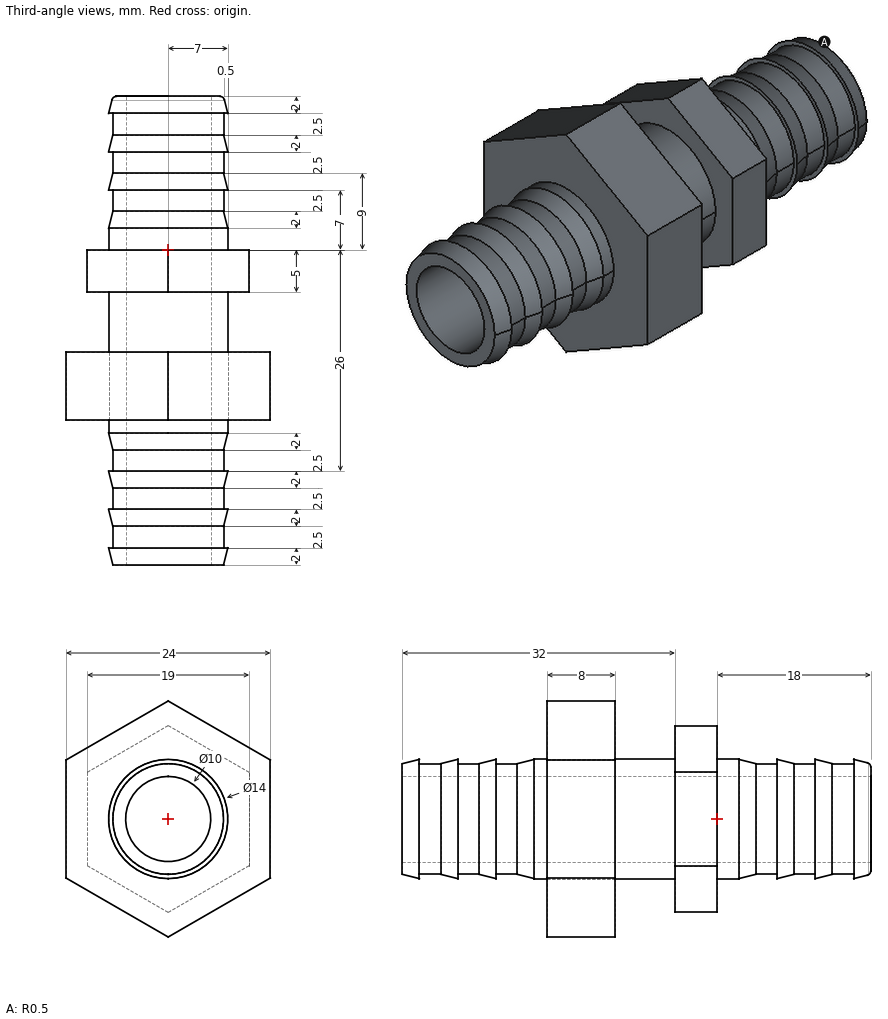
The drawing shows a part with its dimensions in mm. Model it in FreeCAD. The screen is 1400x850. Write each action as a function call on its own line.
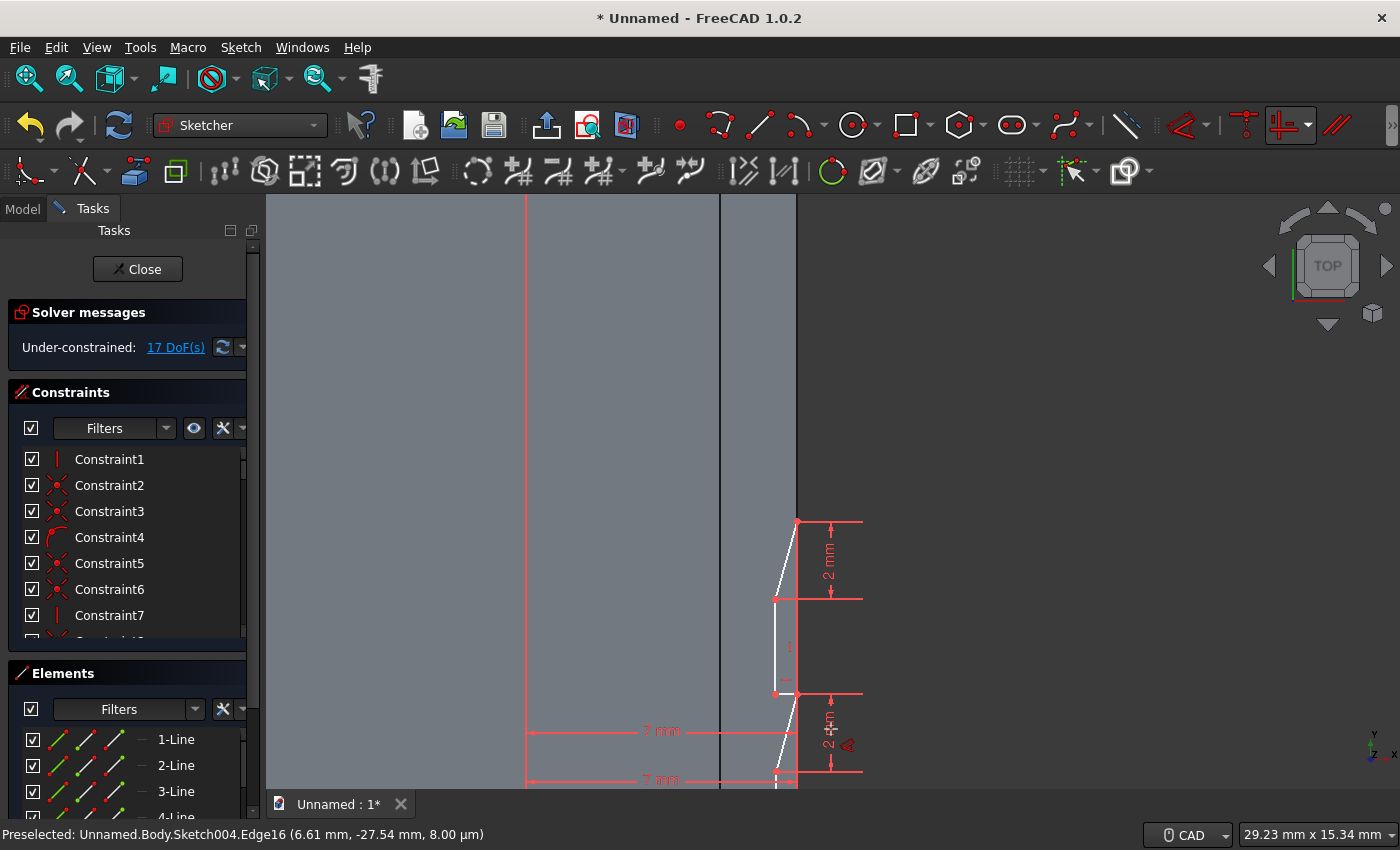
scroll(785, 579, down, 9)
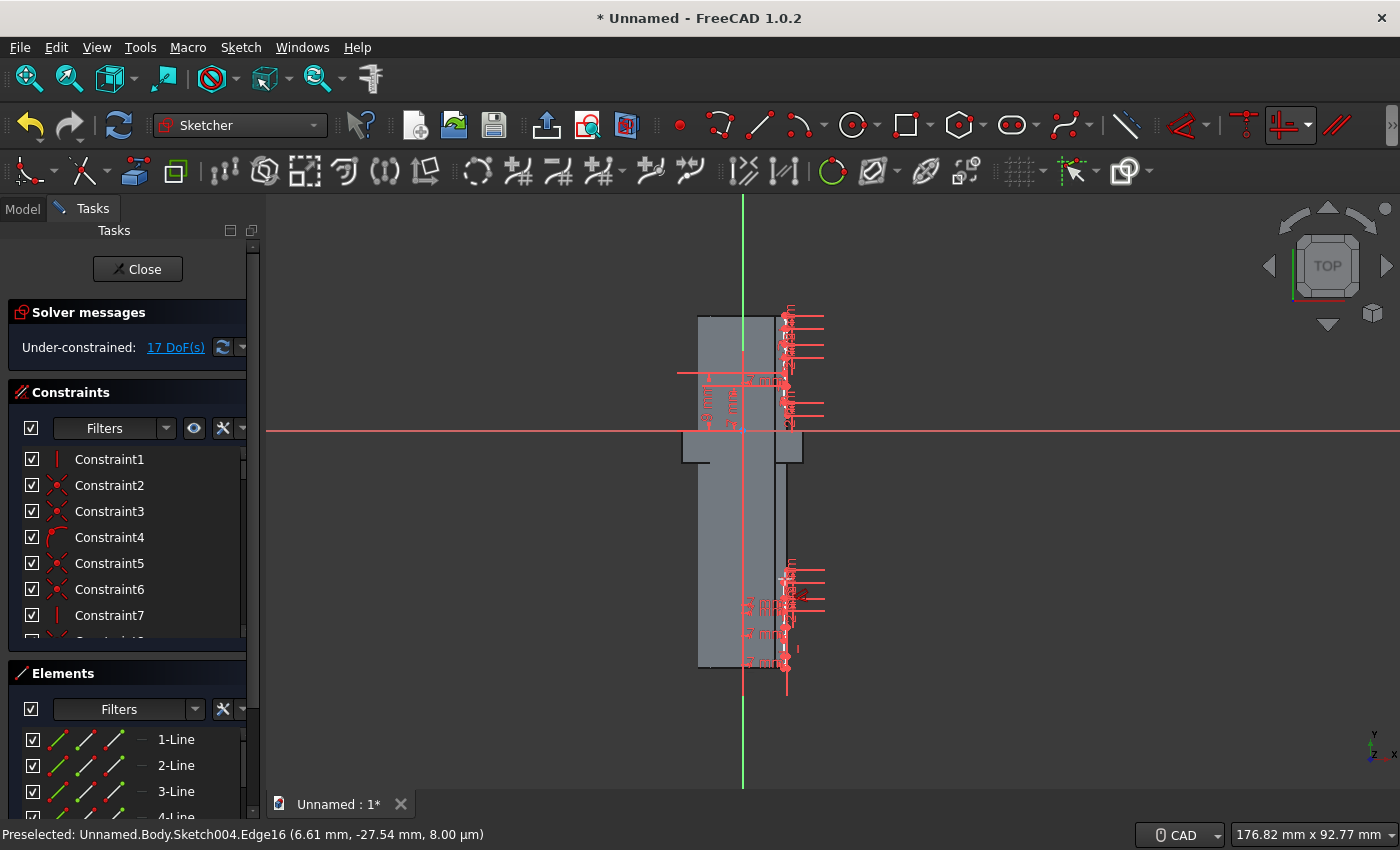
scroll(785, 636, up, 9)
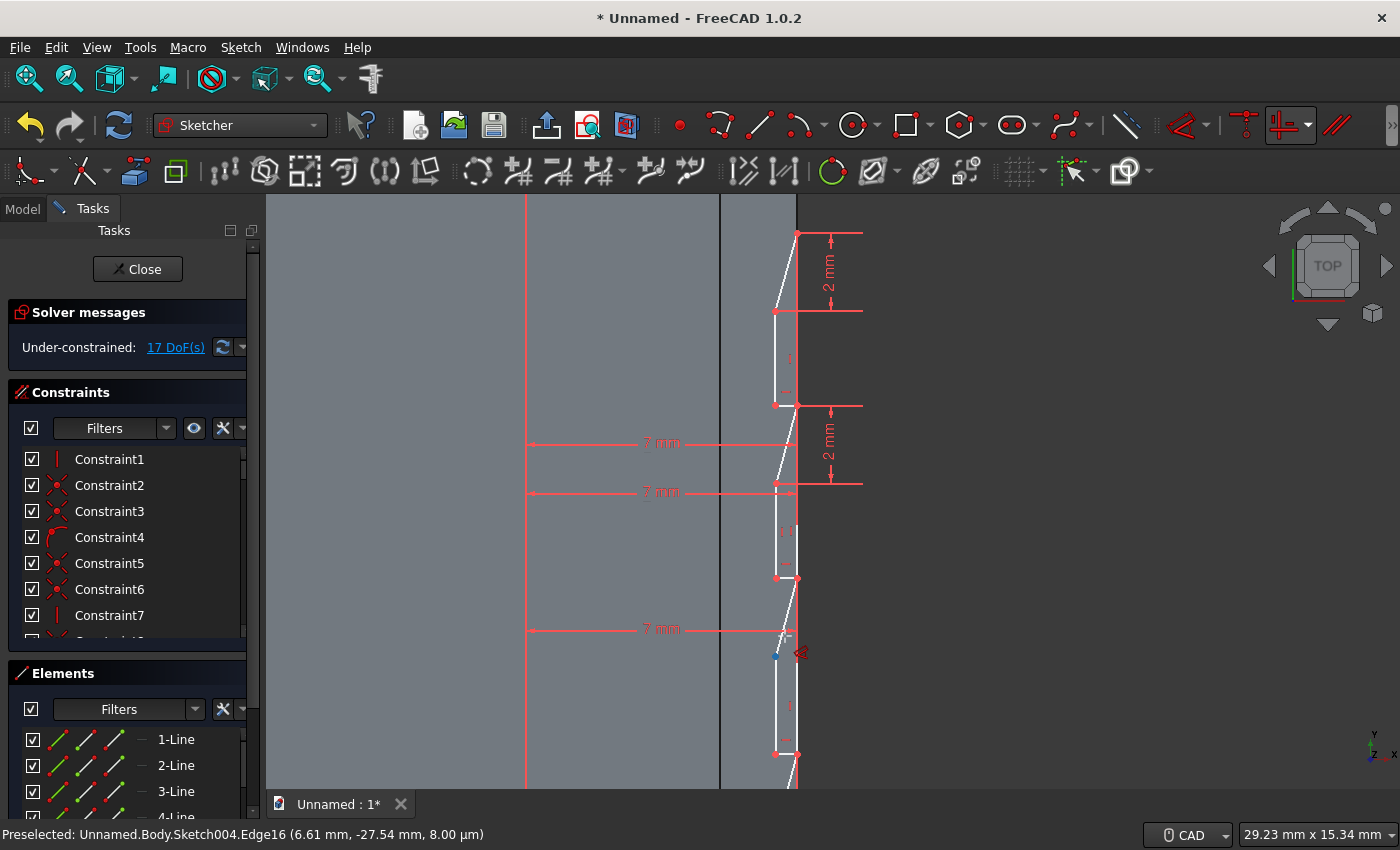
click(782, 633)
click(831, 617)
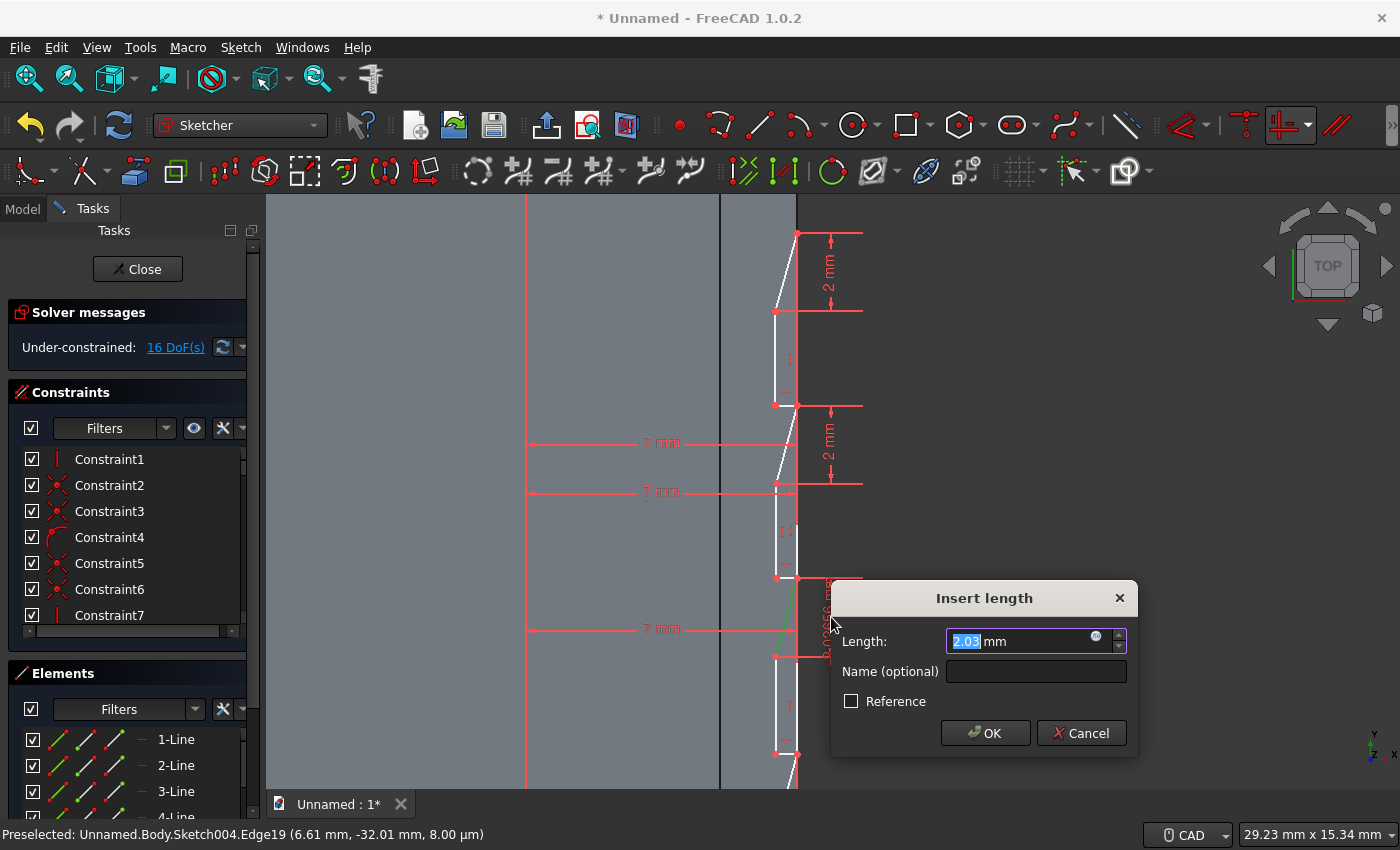
text(2)
key(Return)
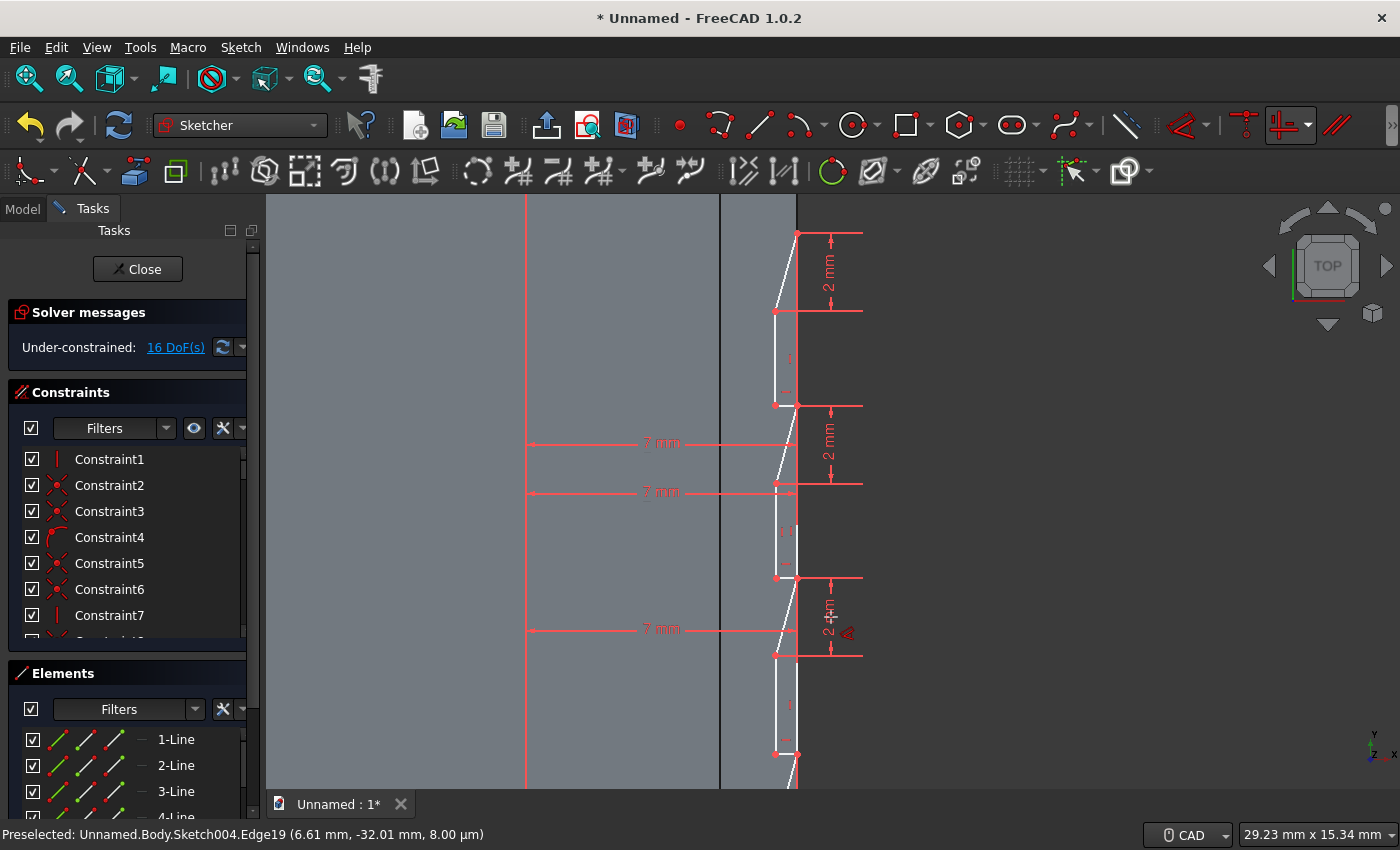
scroll(785, 636, down, 9)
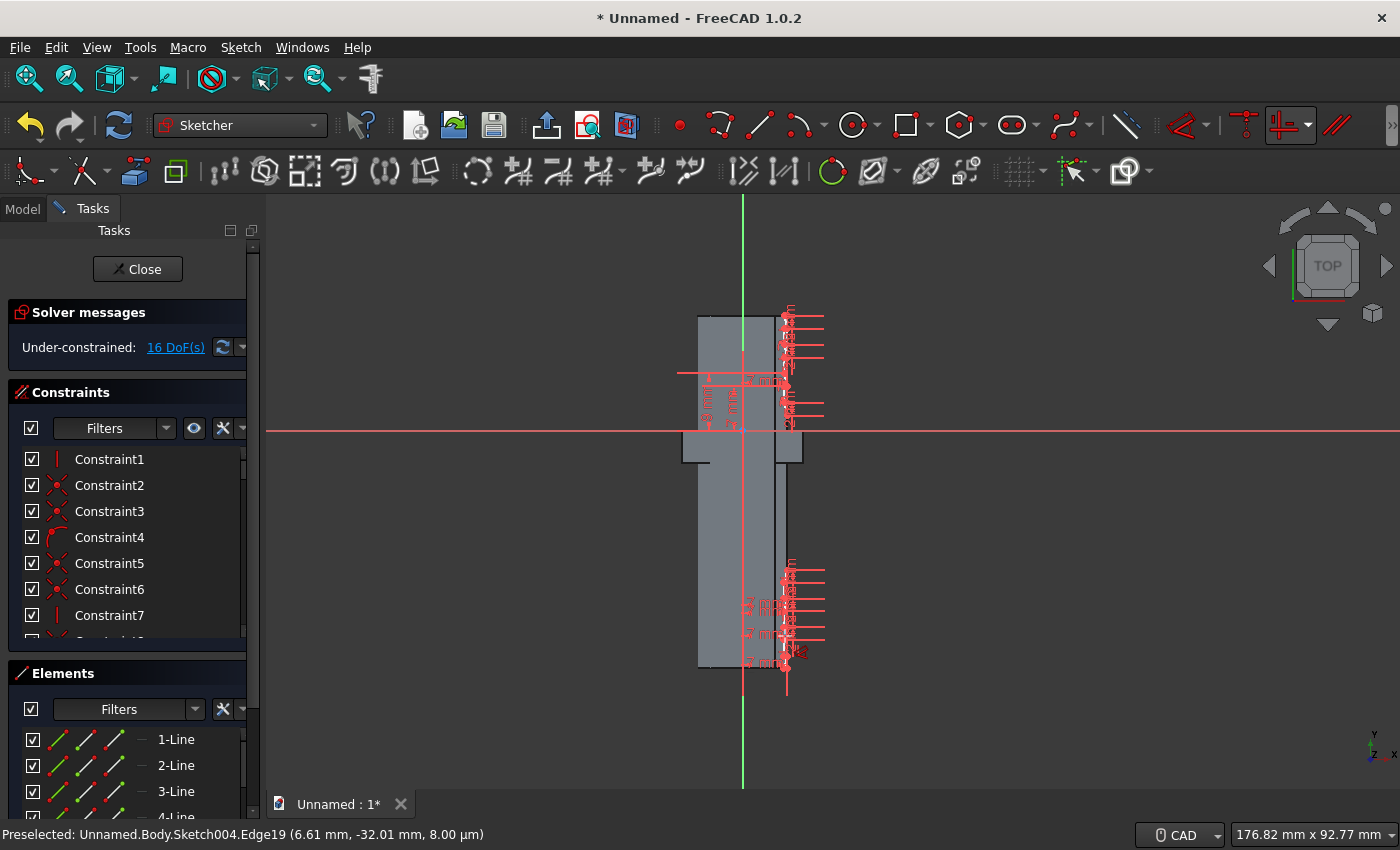
scroll(785, 665, up, 9)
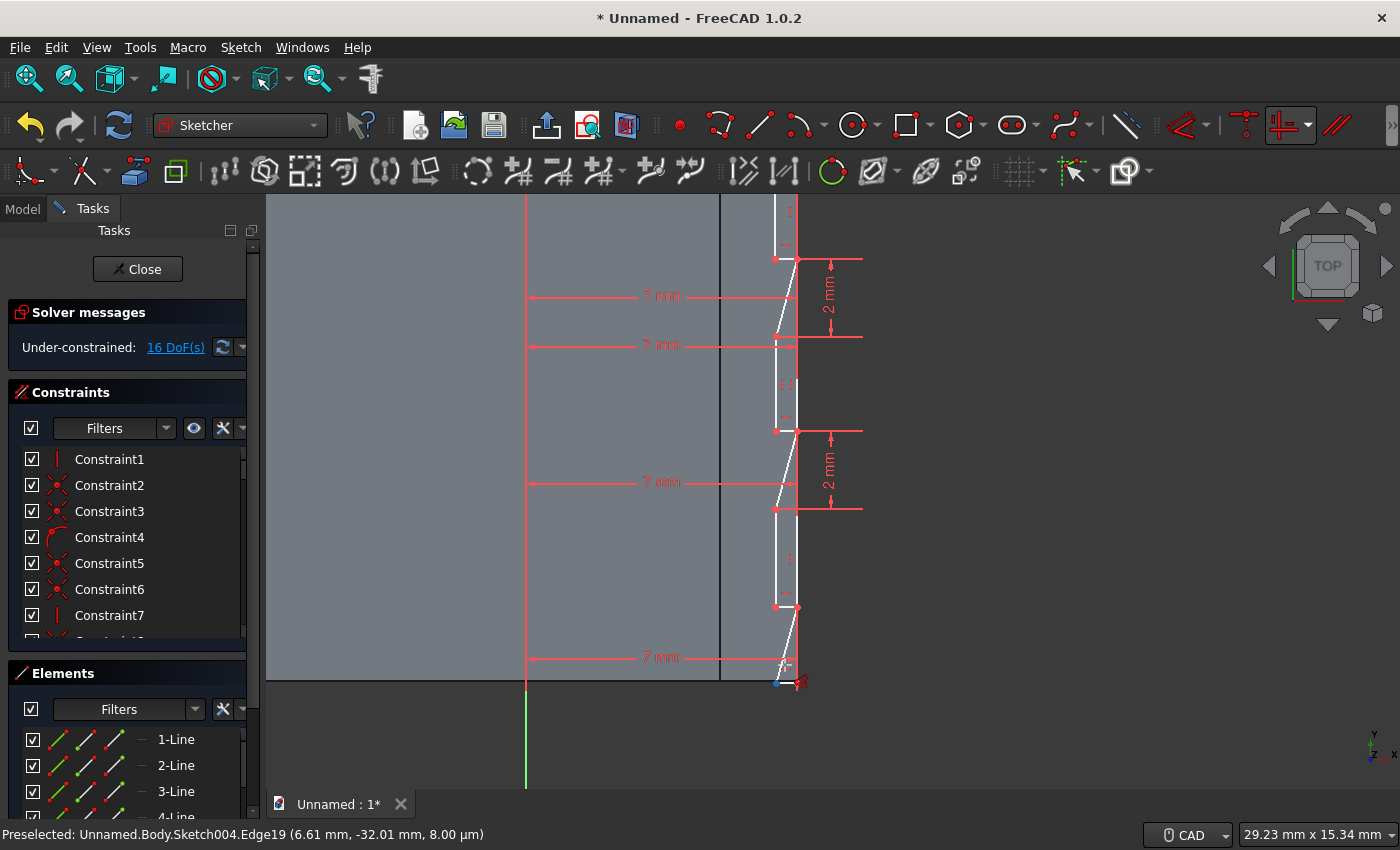
click(783, 660)
click(831, 645)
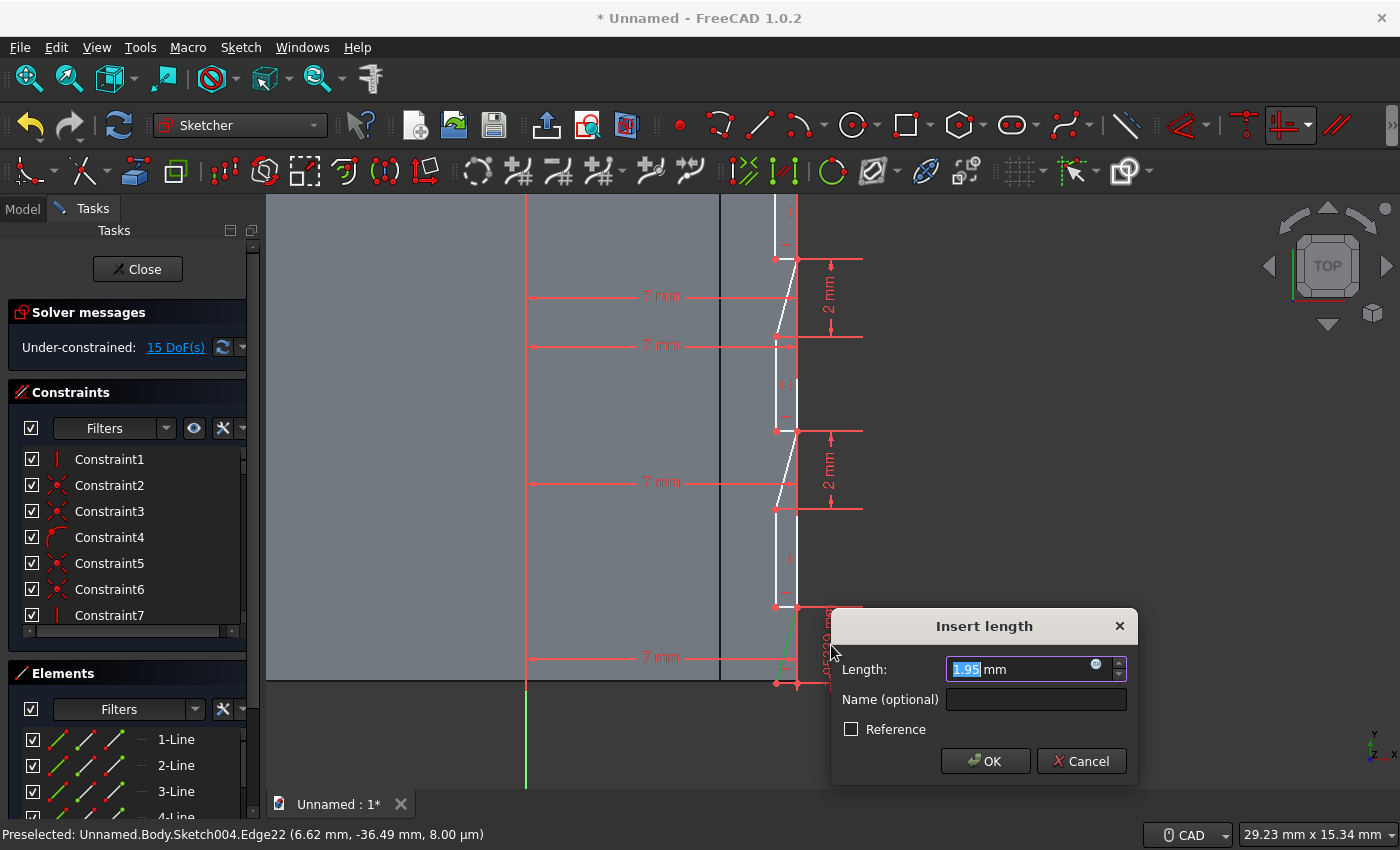
text(2)
key(Return)